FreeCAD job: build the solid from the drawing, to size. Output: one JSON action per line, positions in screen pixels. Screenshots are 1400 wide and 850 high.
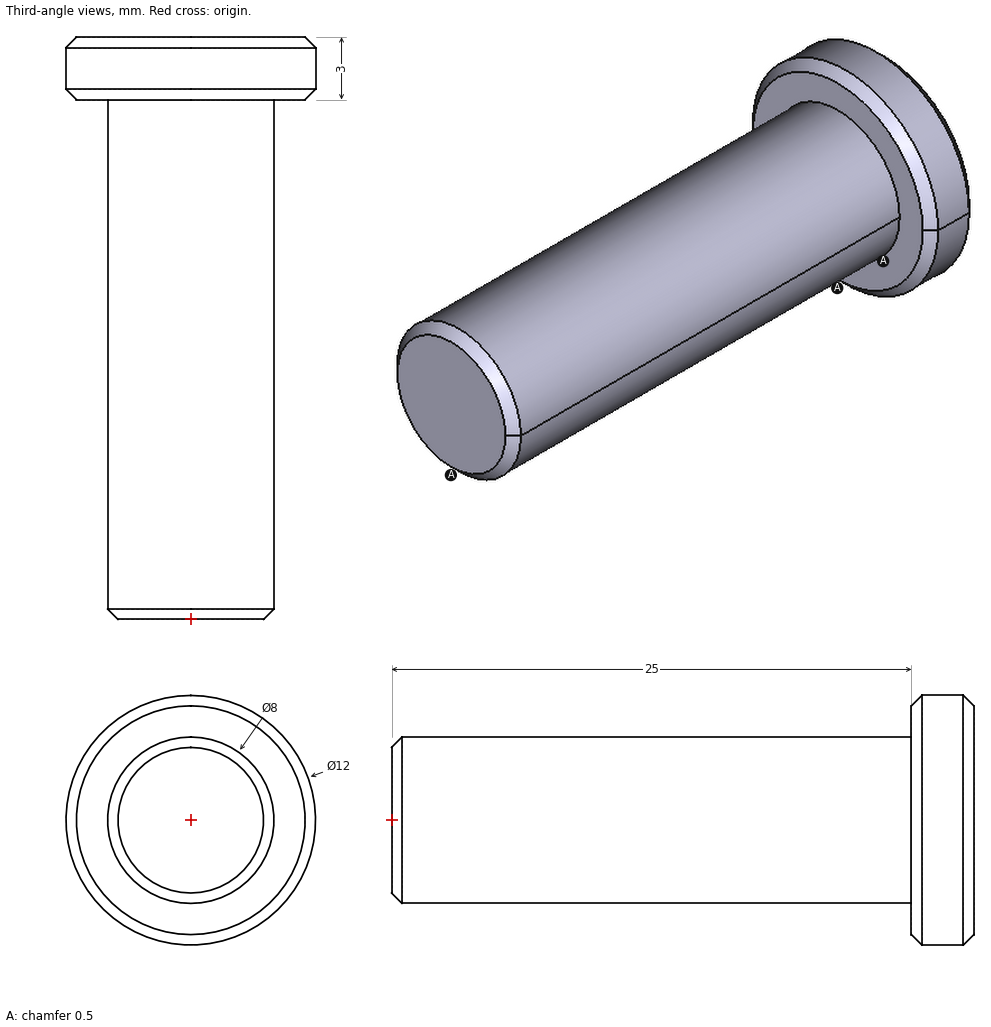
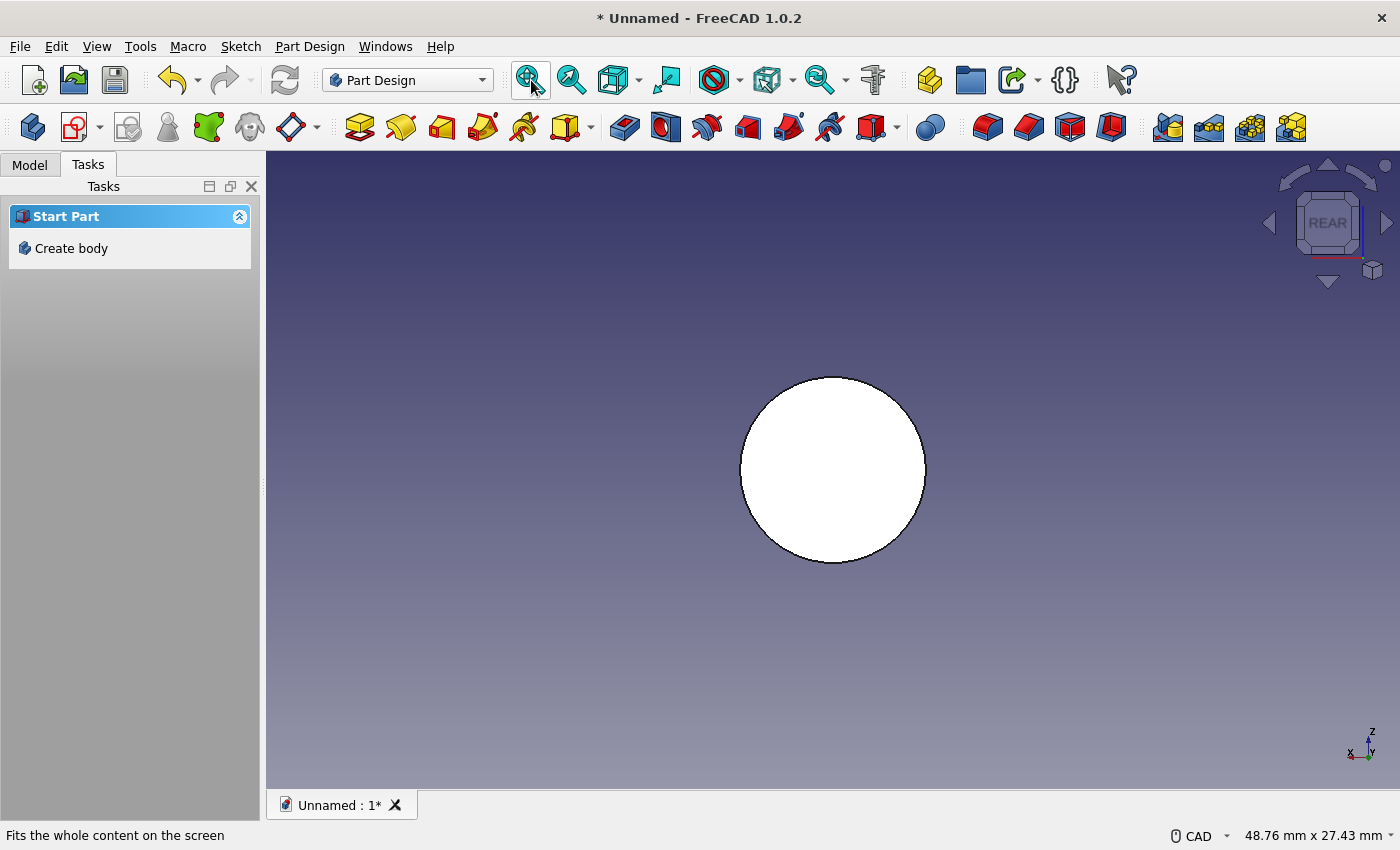
{"action": "left_click", "coordinate": [833, 469]}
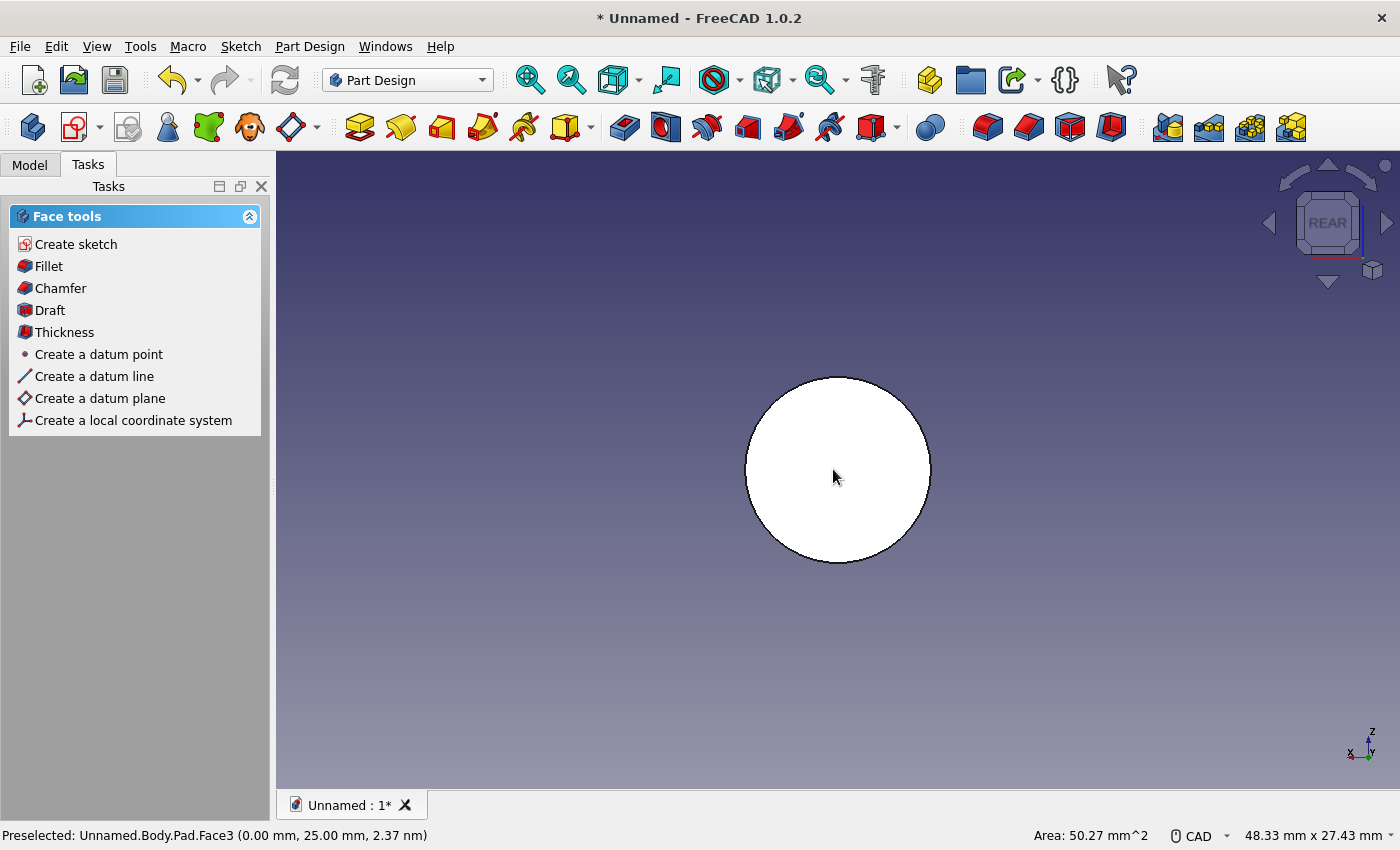
{"action": "left_click", "coordinate": [74, 128]}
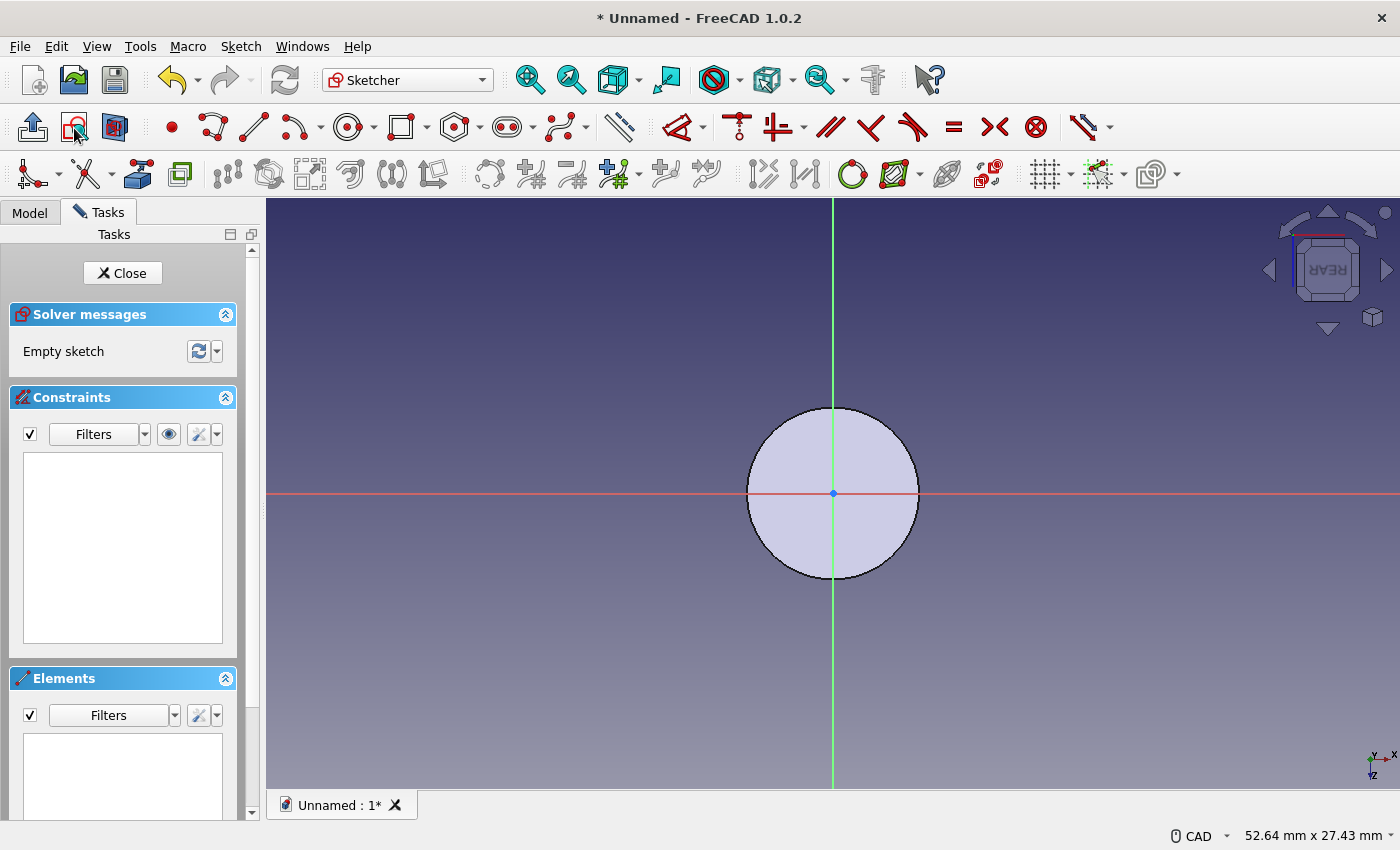
{"action": "scroll", "coordinate": [972, 493], "scroll_direction": "up", "scroll_amount": 2}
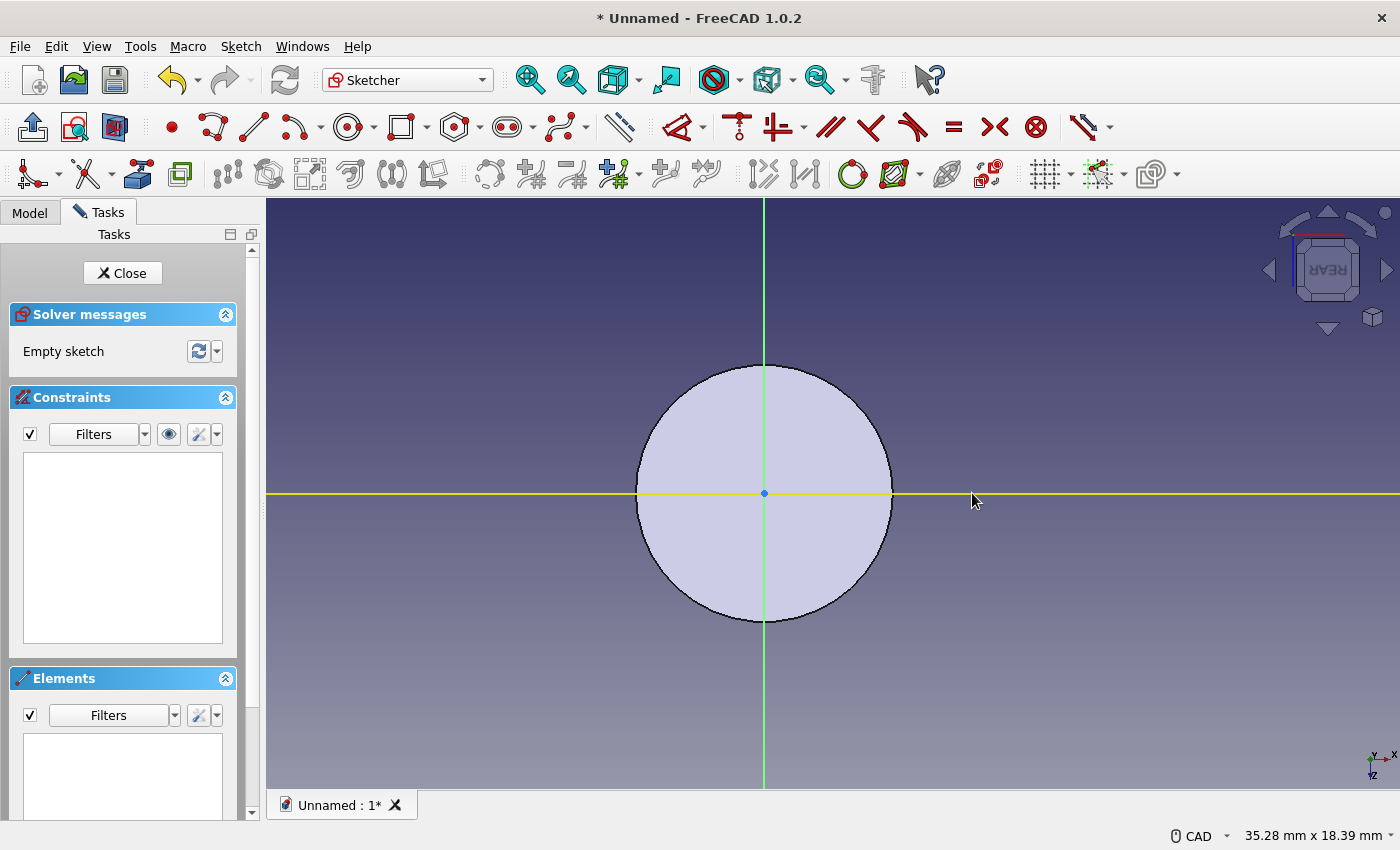
{"action": "key", "text": "g c"}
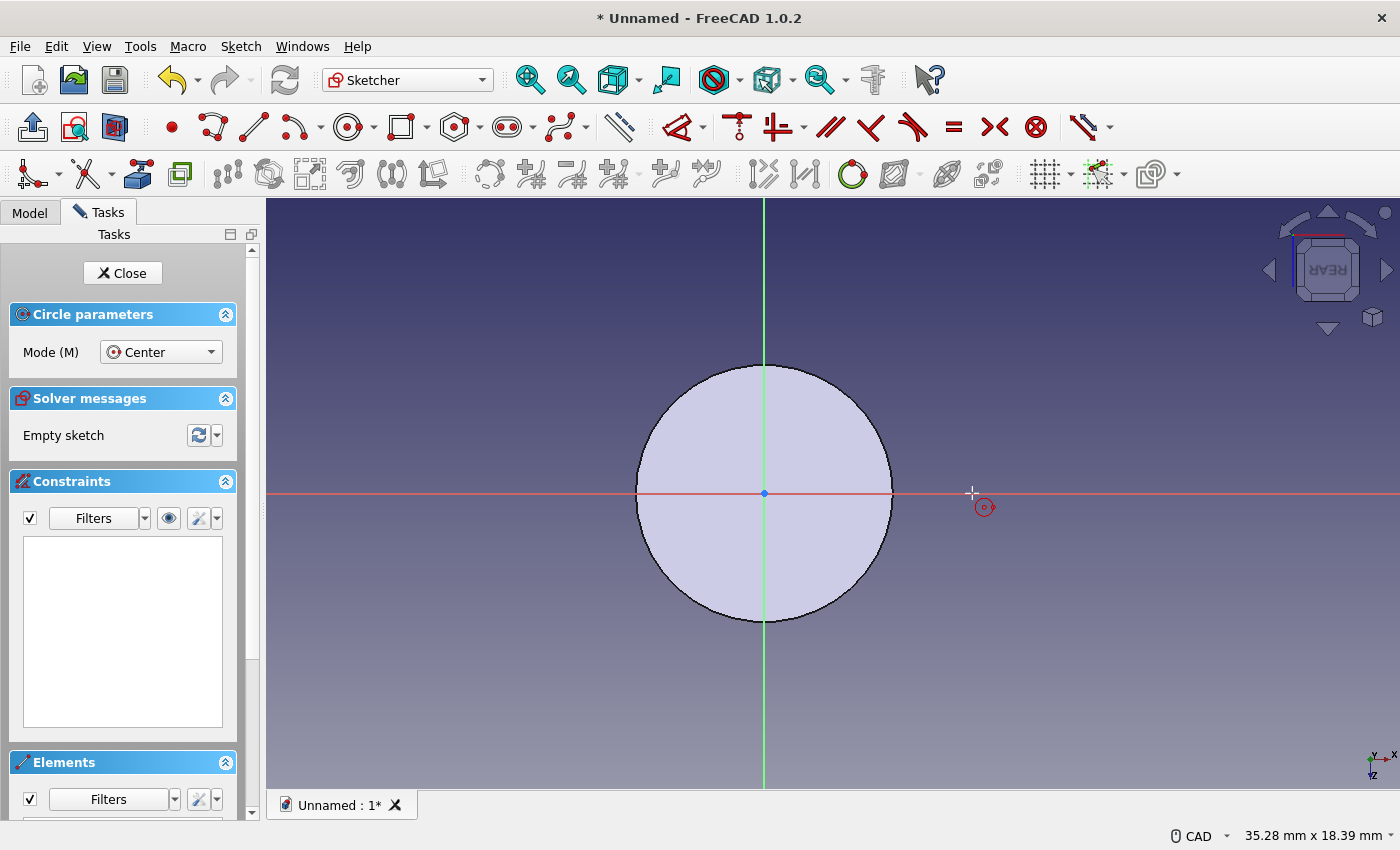
{"action": "left_click", "coordinate": [764, 493]}
{"action": "mouse_move", "coordinate": [901, 357]}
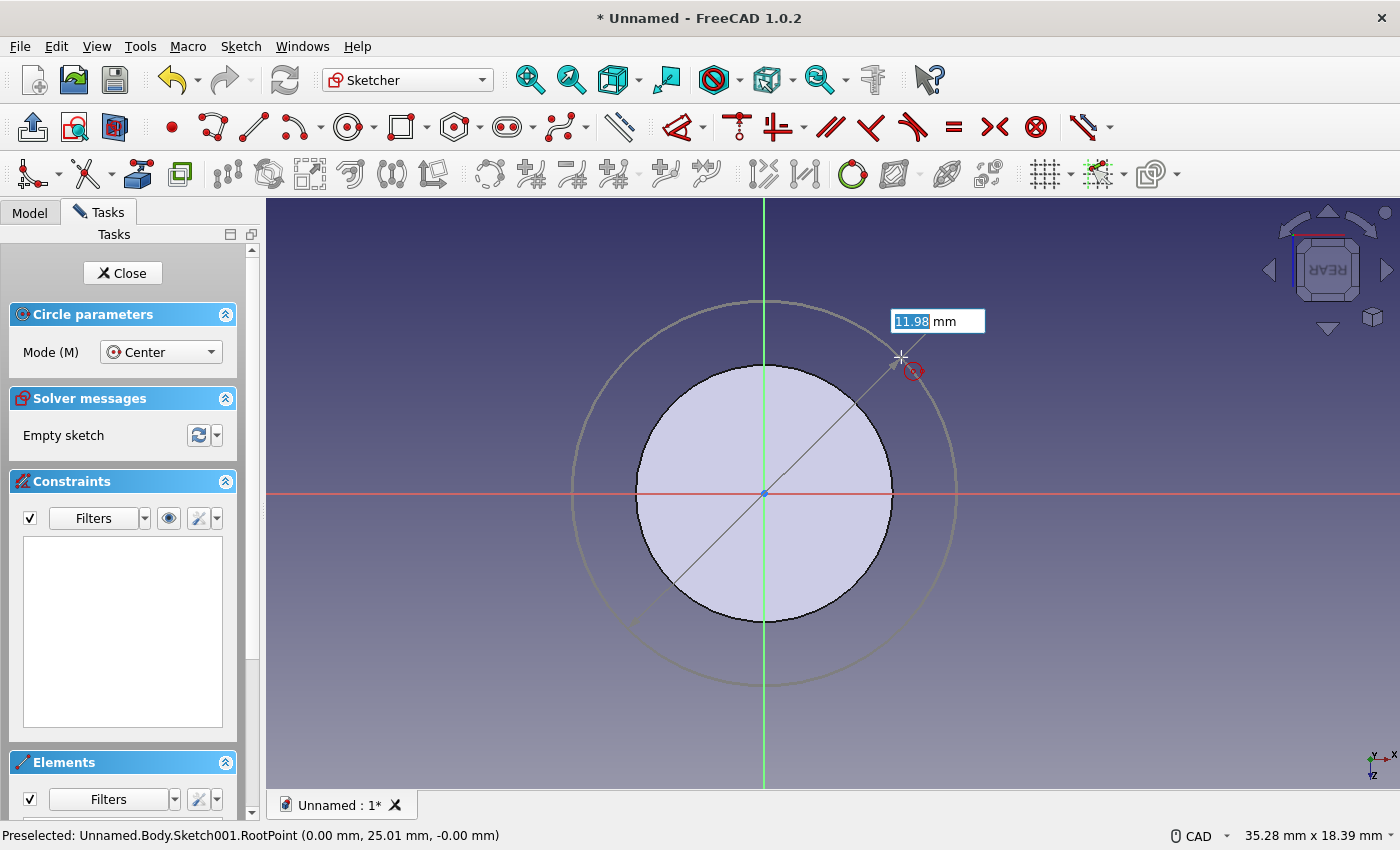
{"action": "type", "text": "12"}
{"action": "key", "text": "Return"}
{"action": "key", "text": "Escape"}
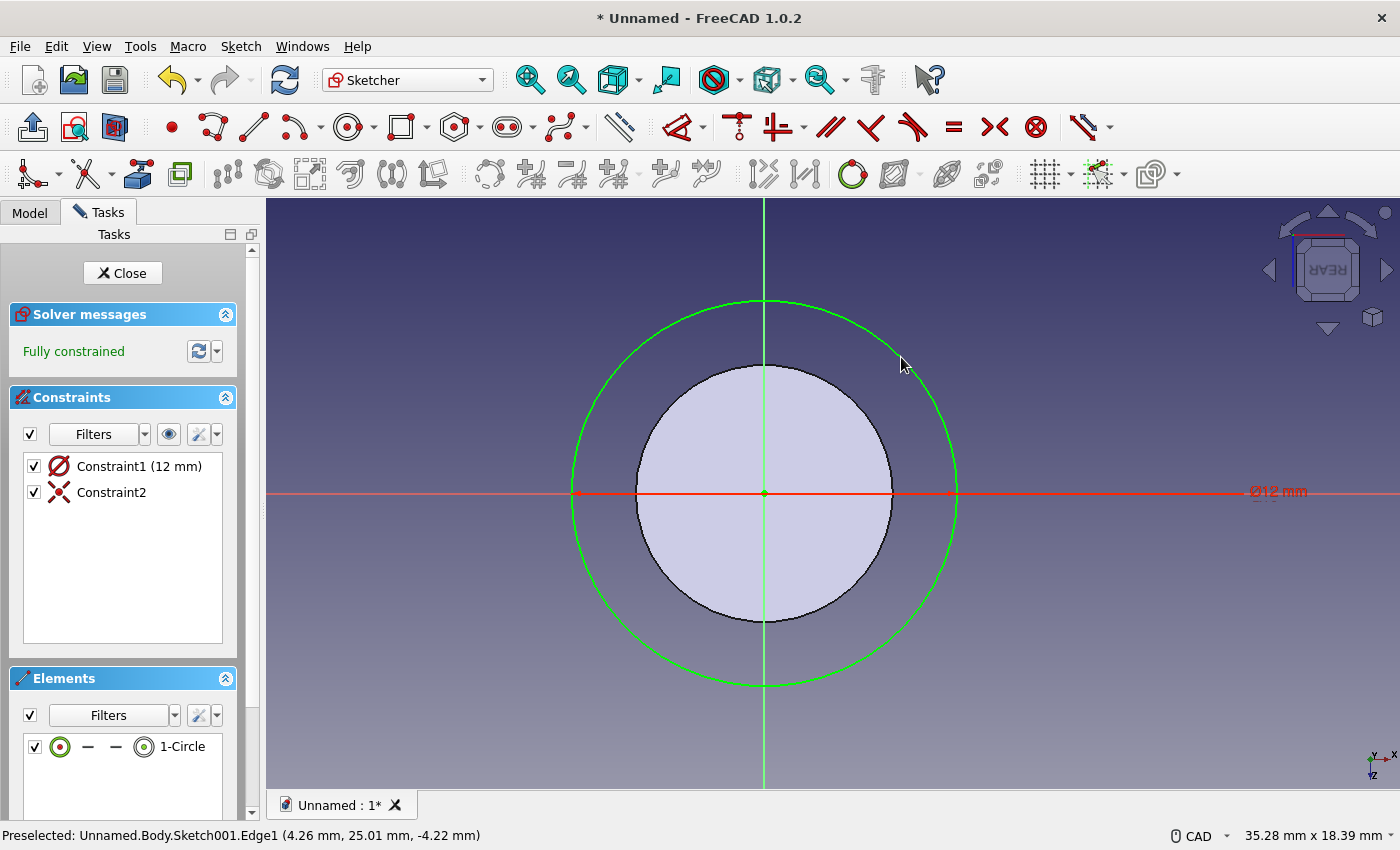
{"action": "left_click", "coordinate": [123, 273]}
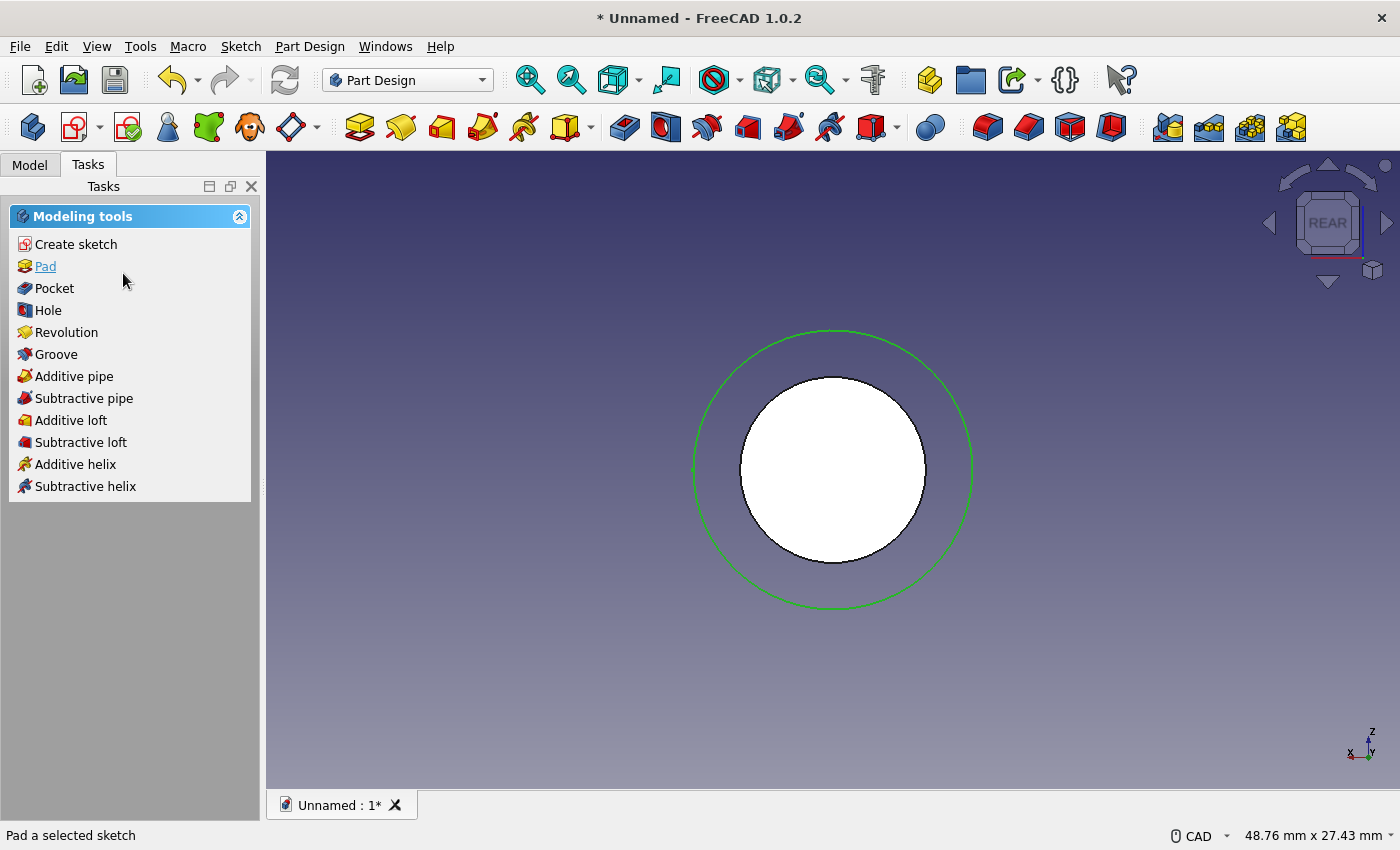
{"action": "left_click", "coordinate": [360, 128]}